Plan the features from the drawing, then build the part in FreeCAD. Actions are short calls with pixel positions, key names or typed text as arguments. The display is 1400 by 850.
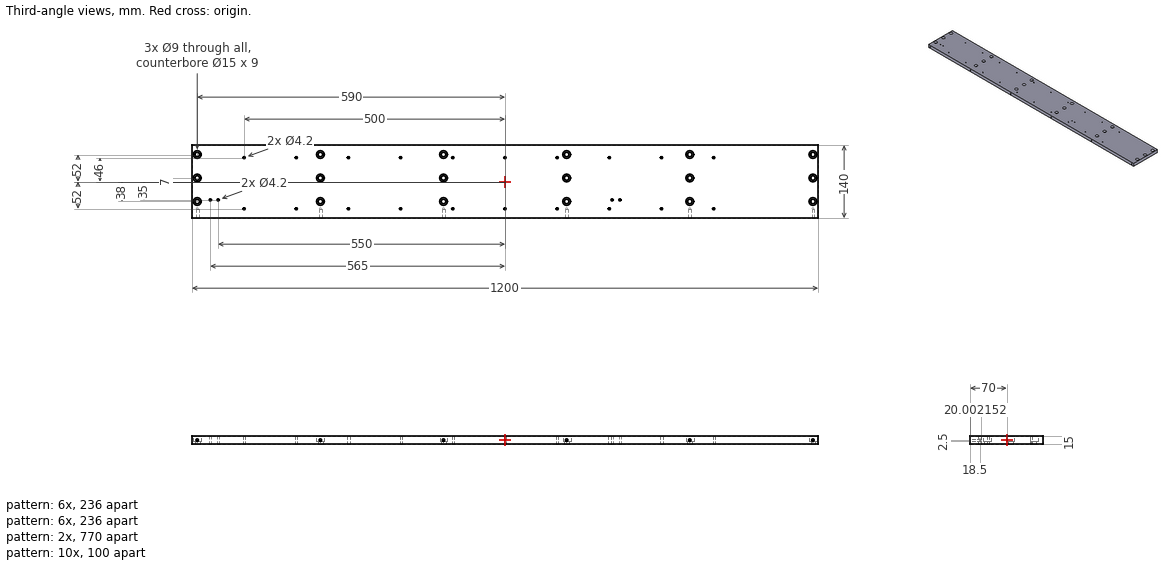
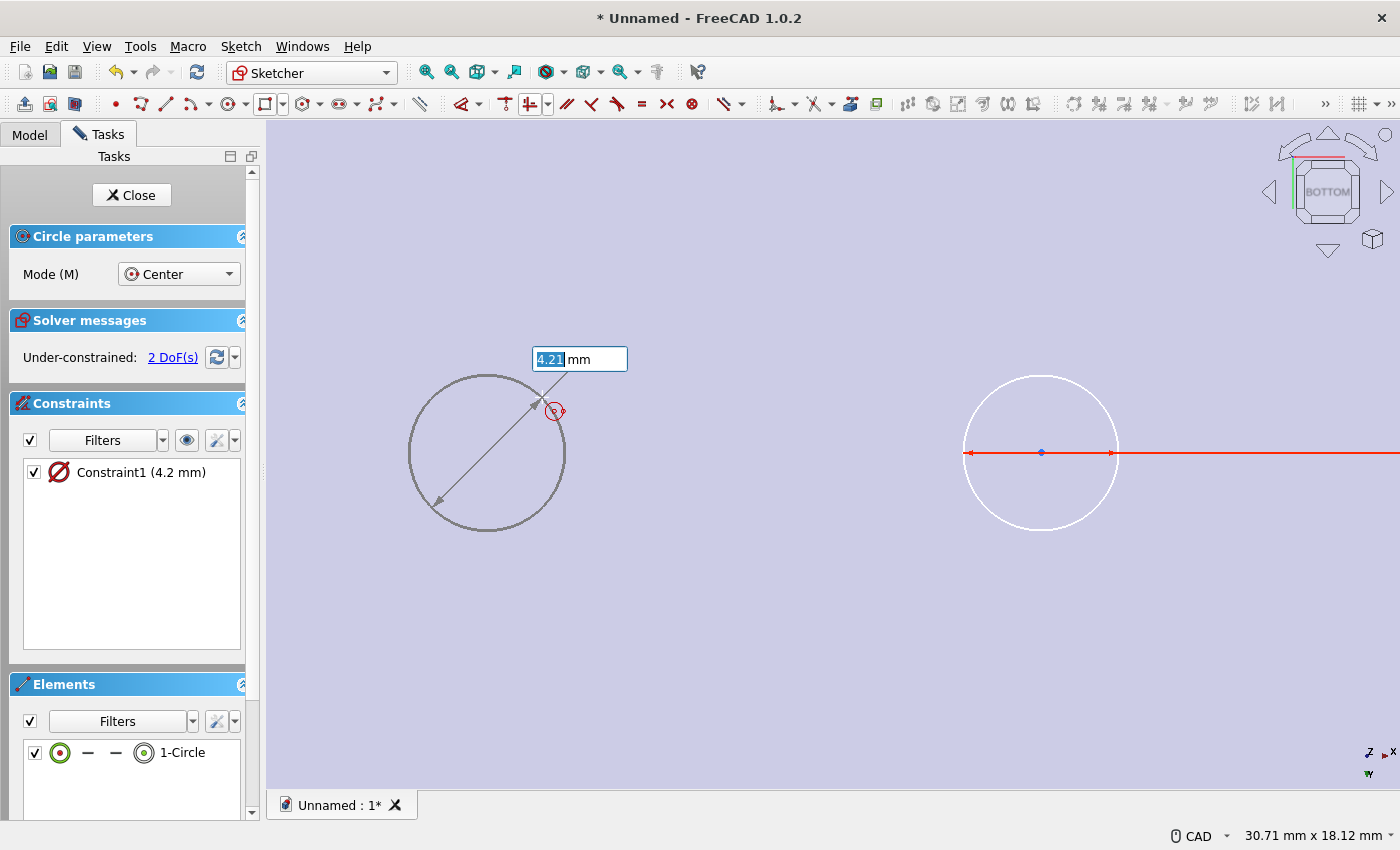
text(4.2)
key(Return)
key(Escape)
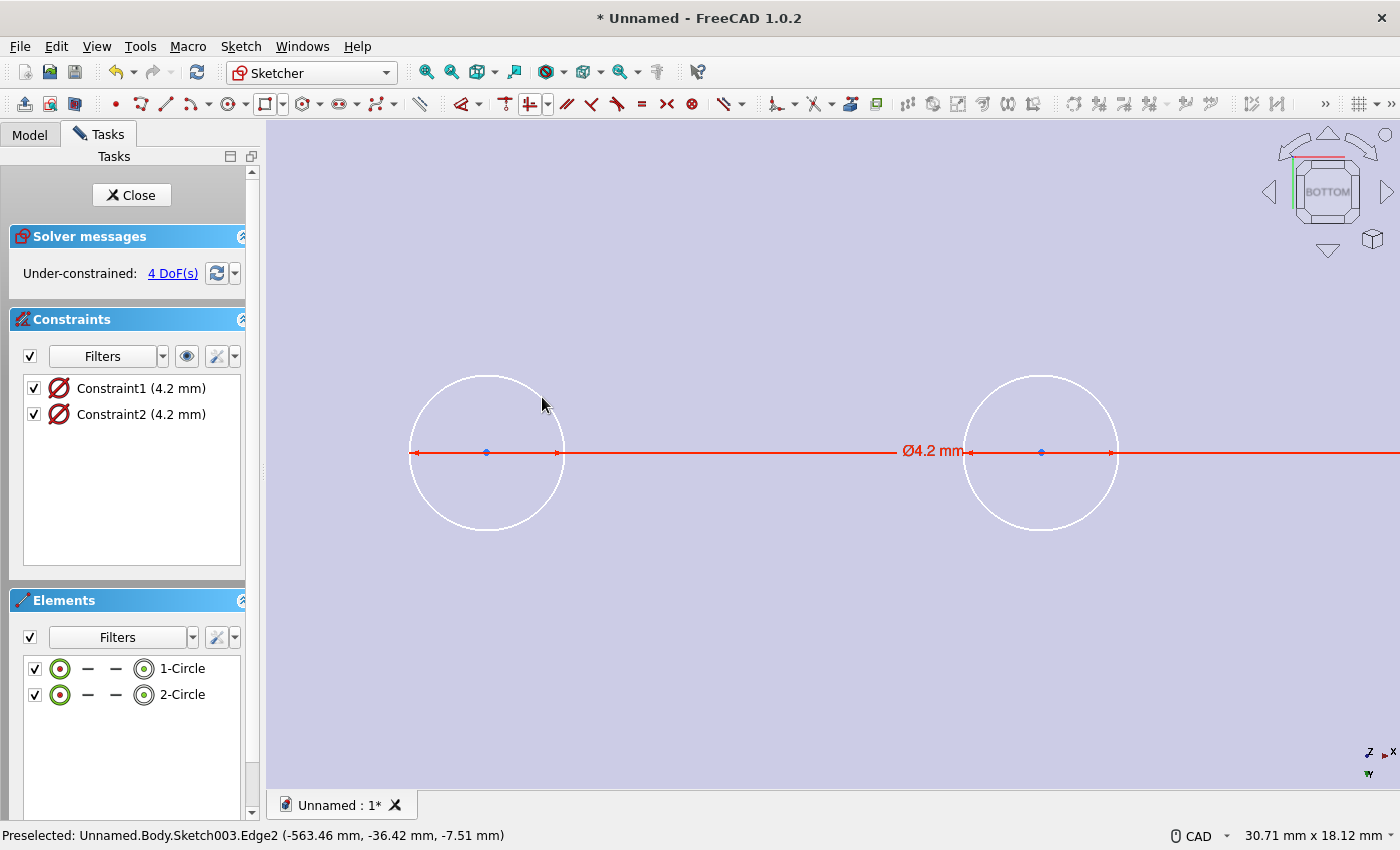
click(1041, 453)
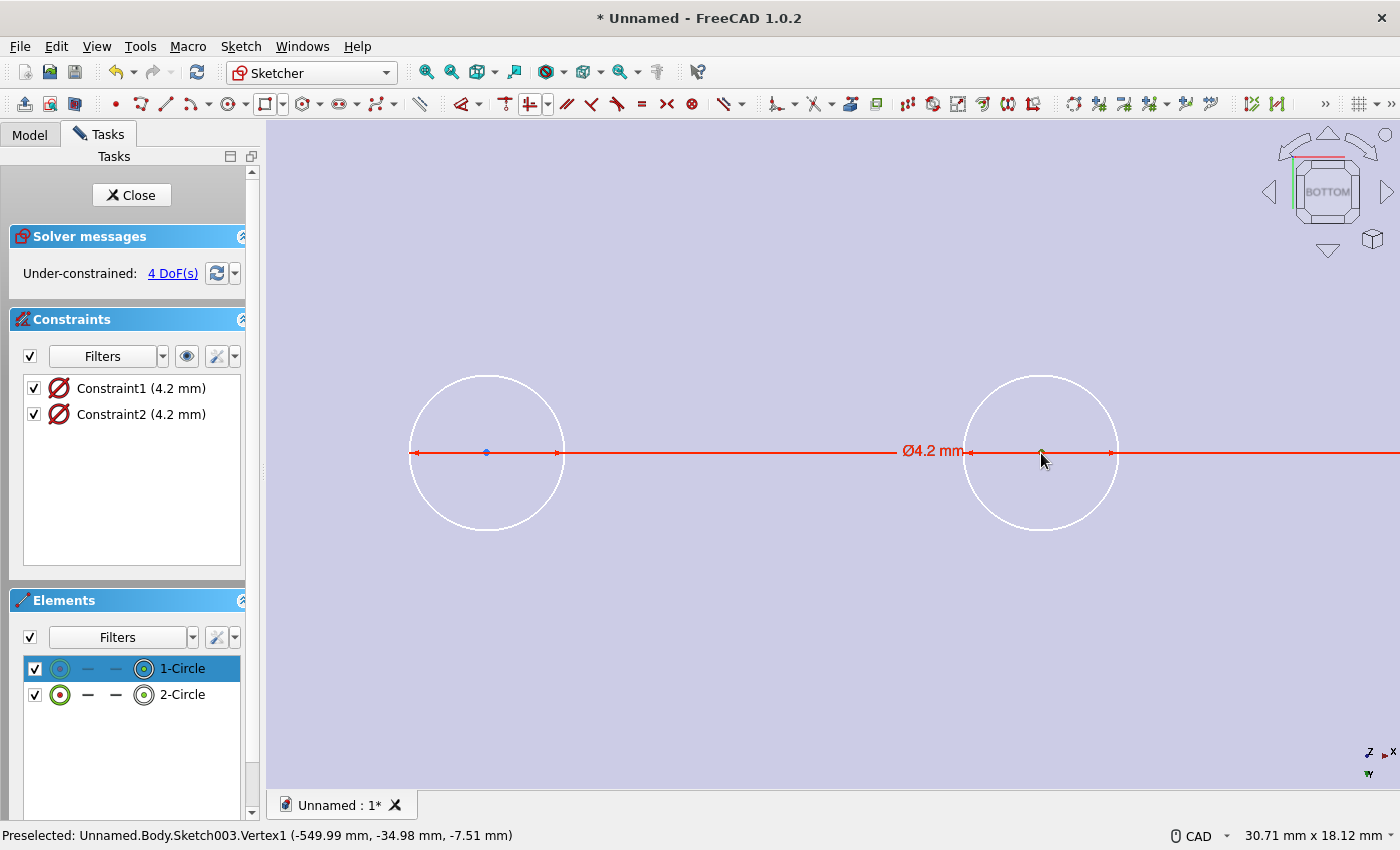
click(487, 453)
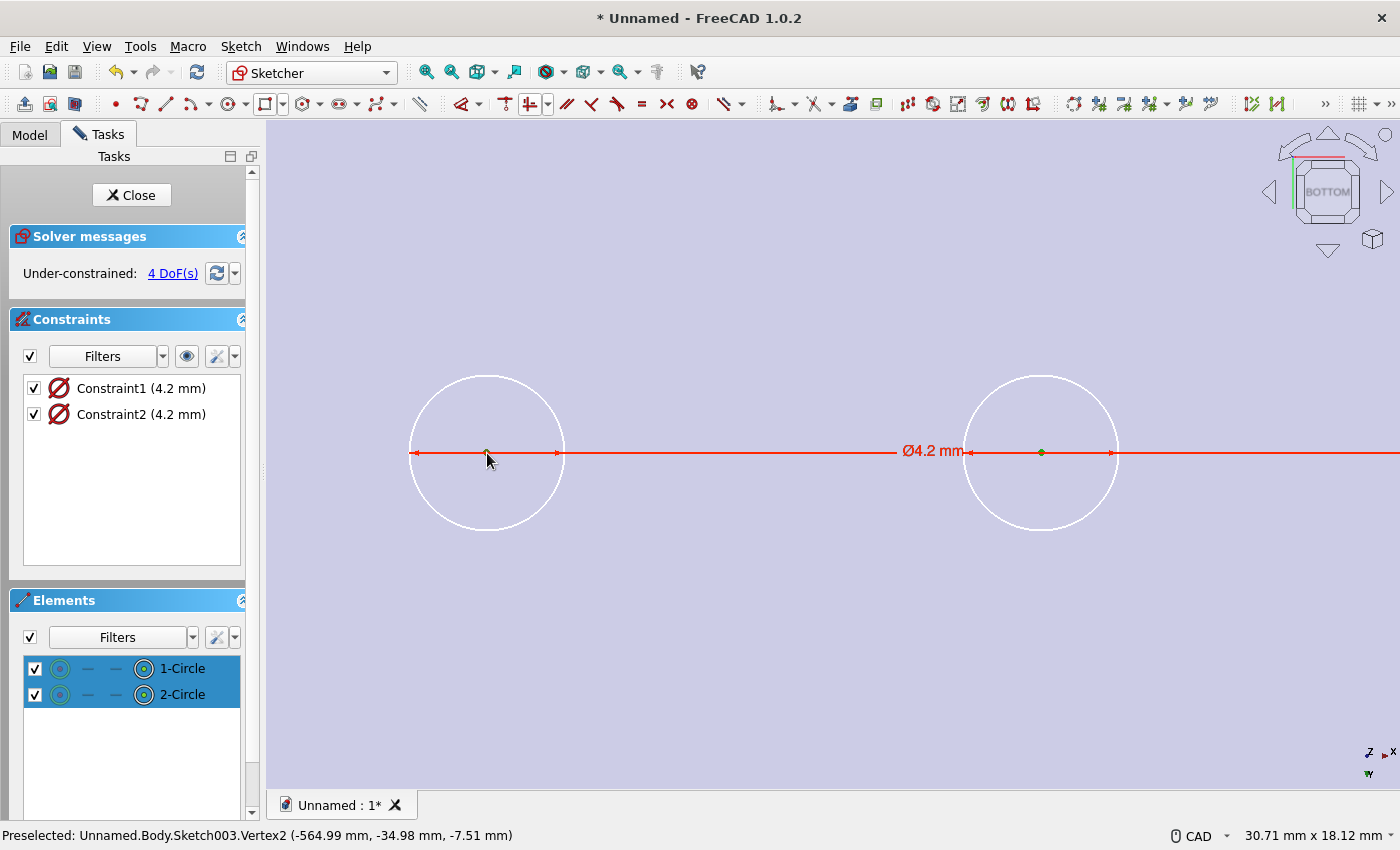
key(h)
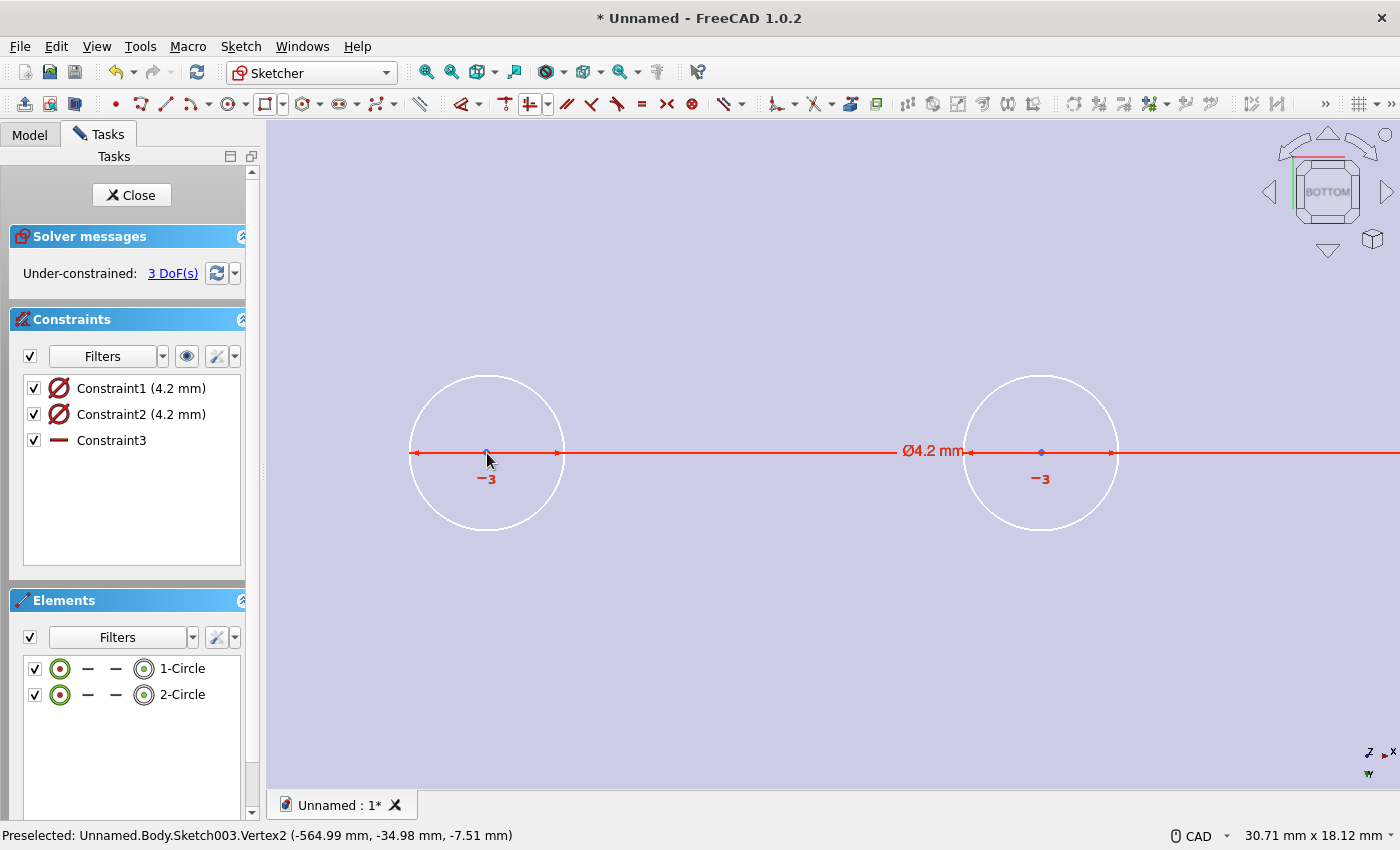
key(d)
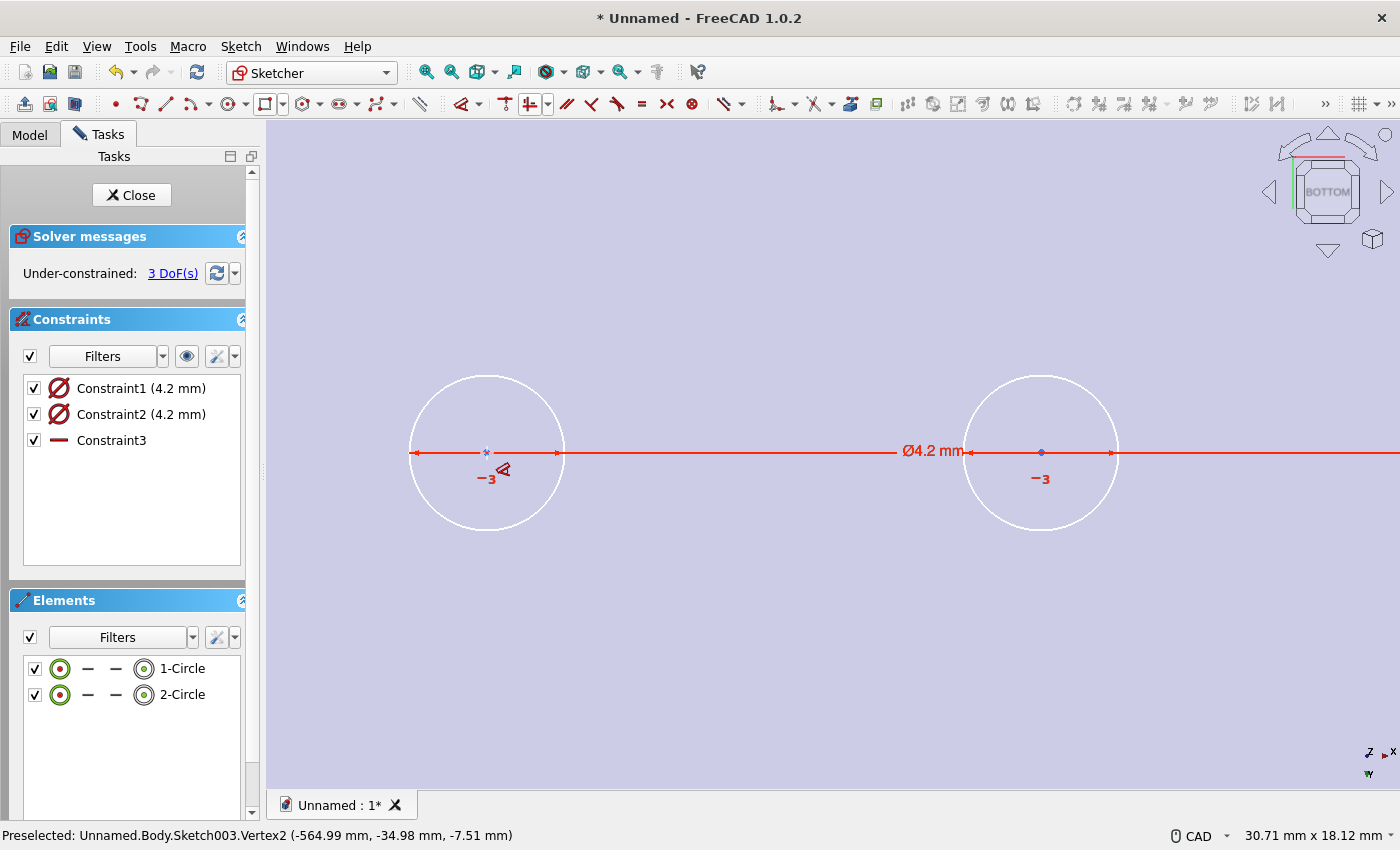
click(1041, 453)
click(1007, 607)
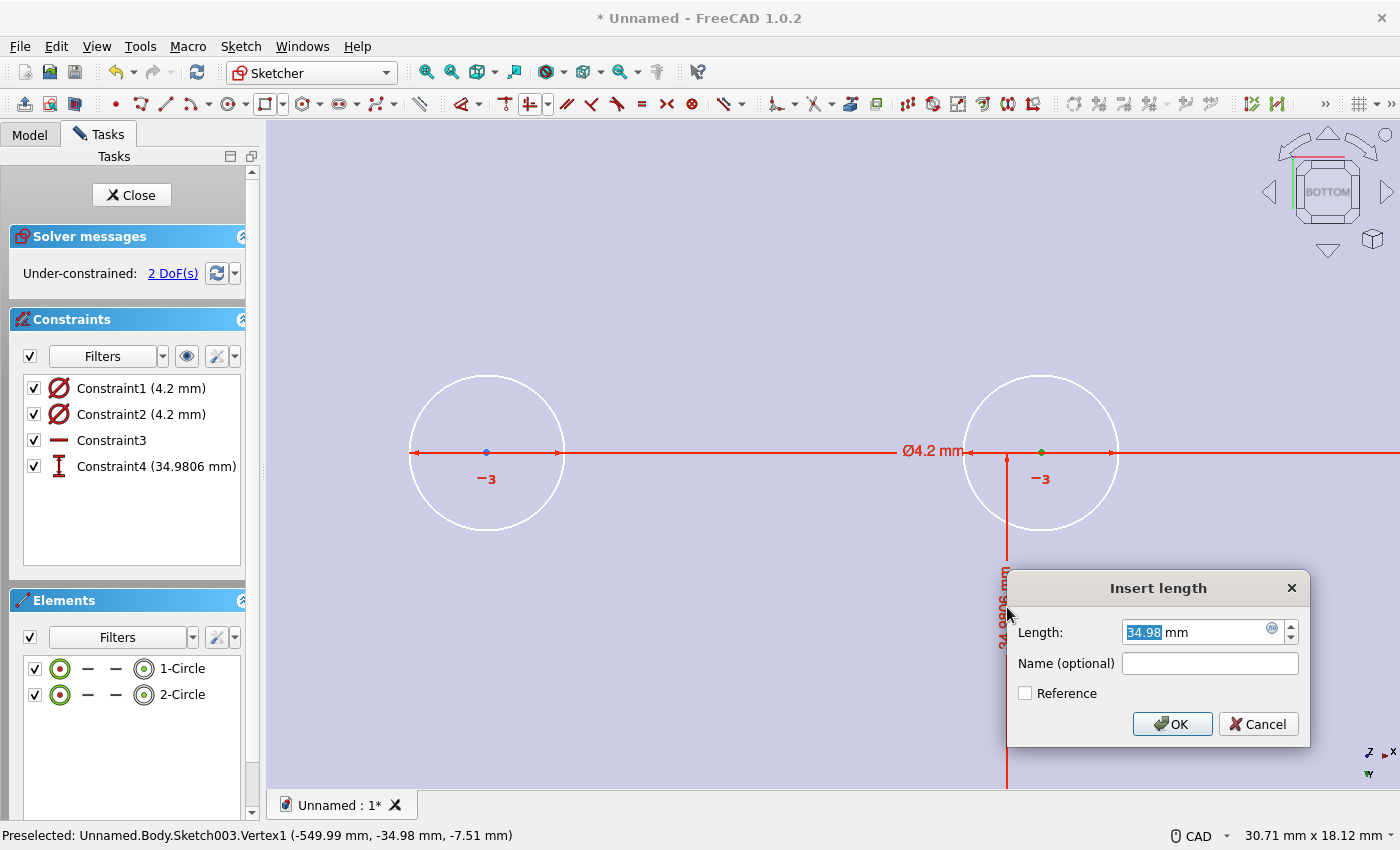
text(35)
key(Return)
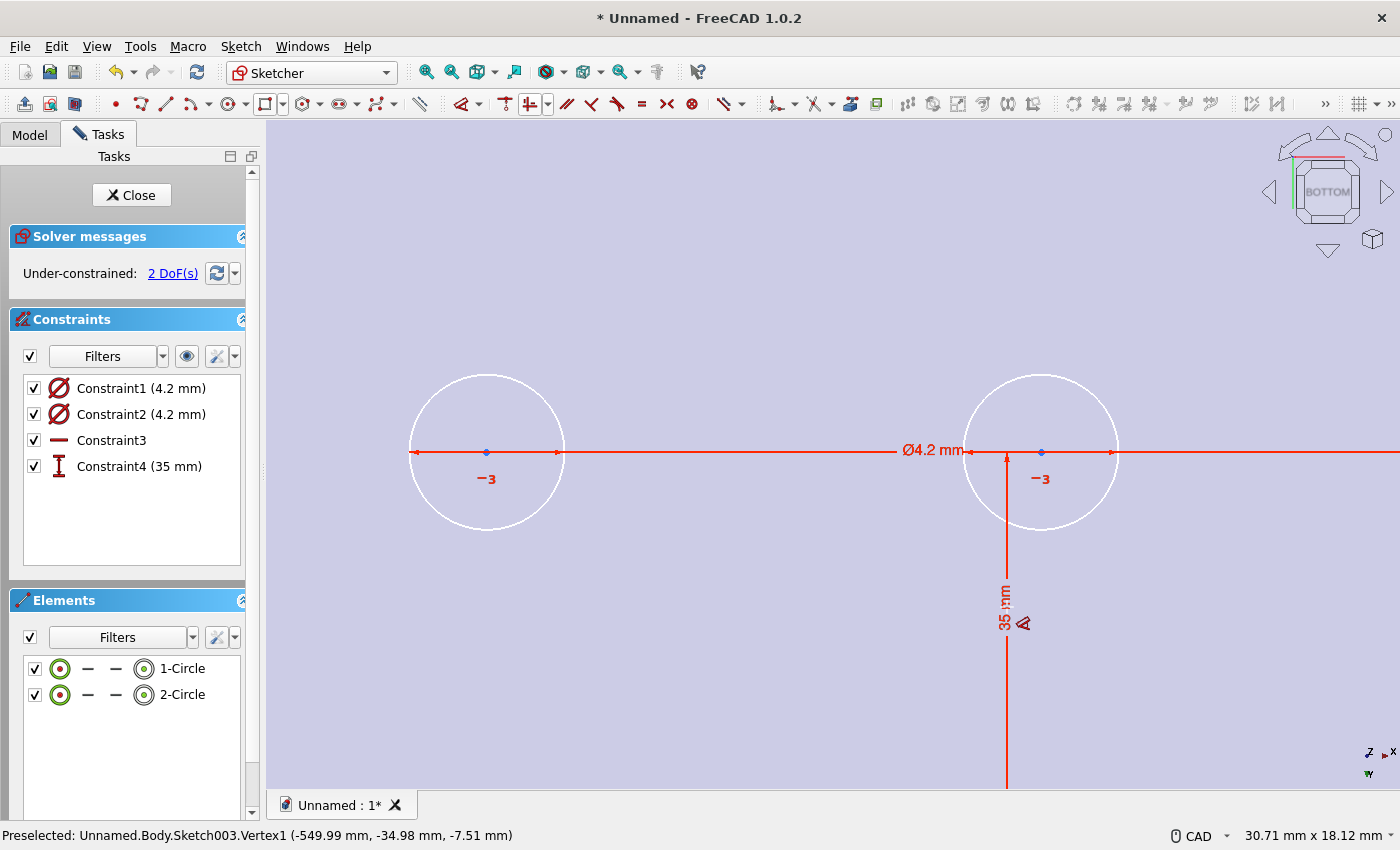
click(1041, 452)
click(1138, 418)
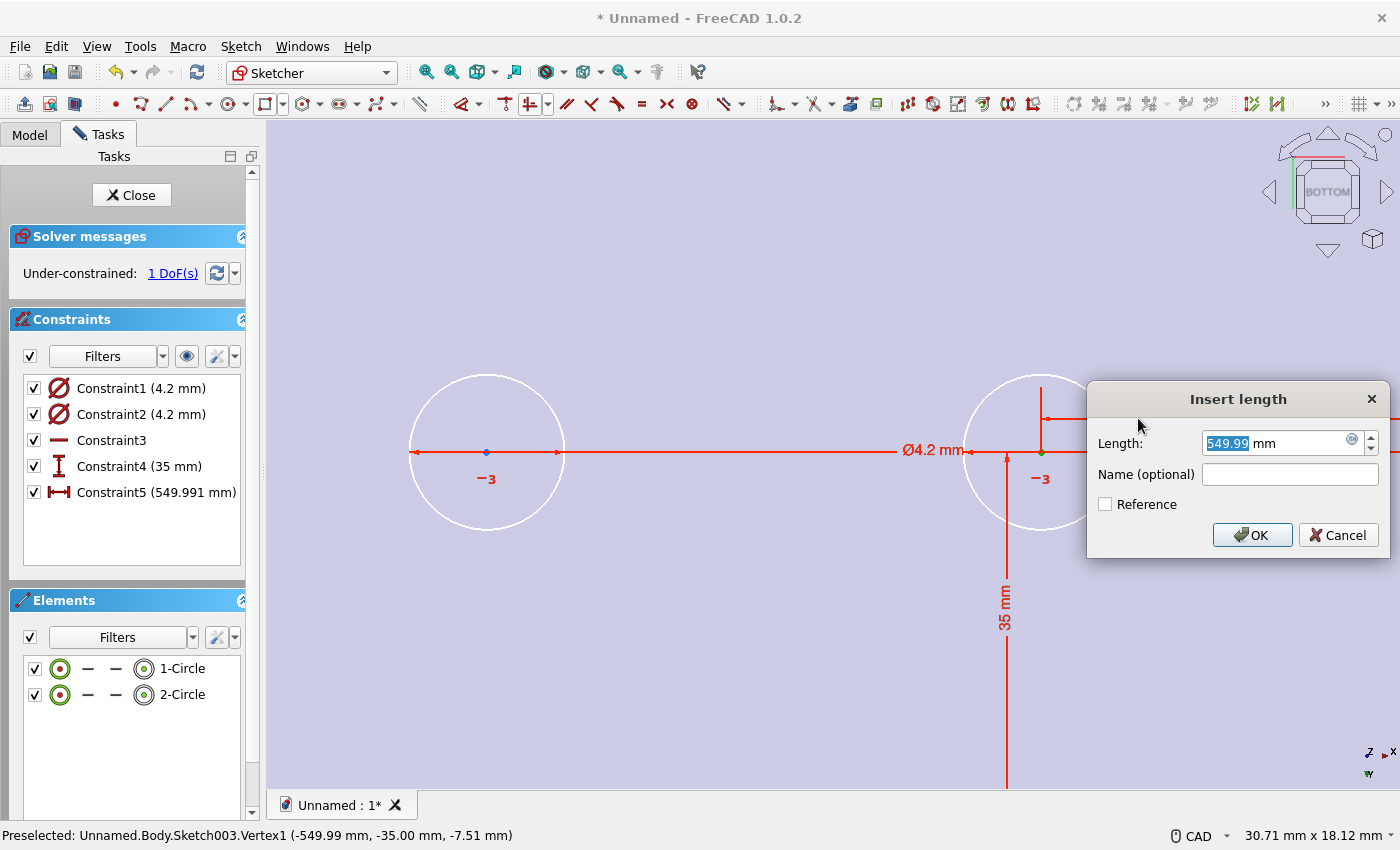
text(550)
key(Return)